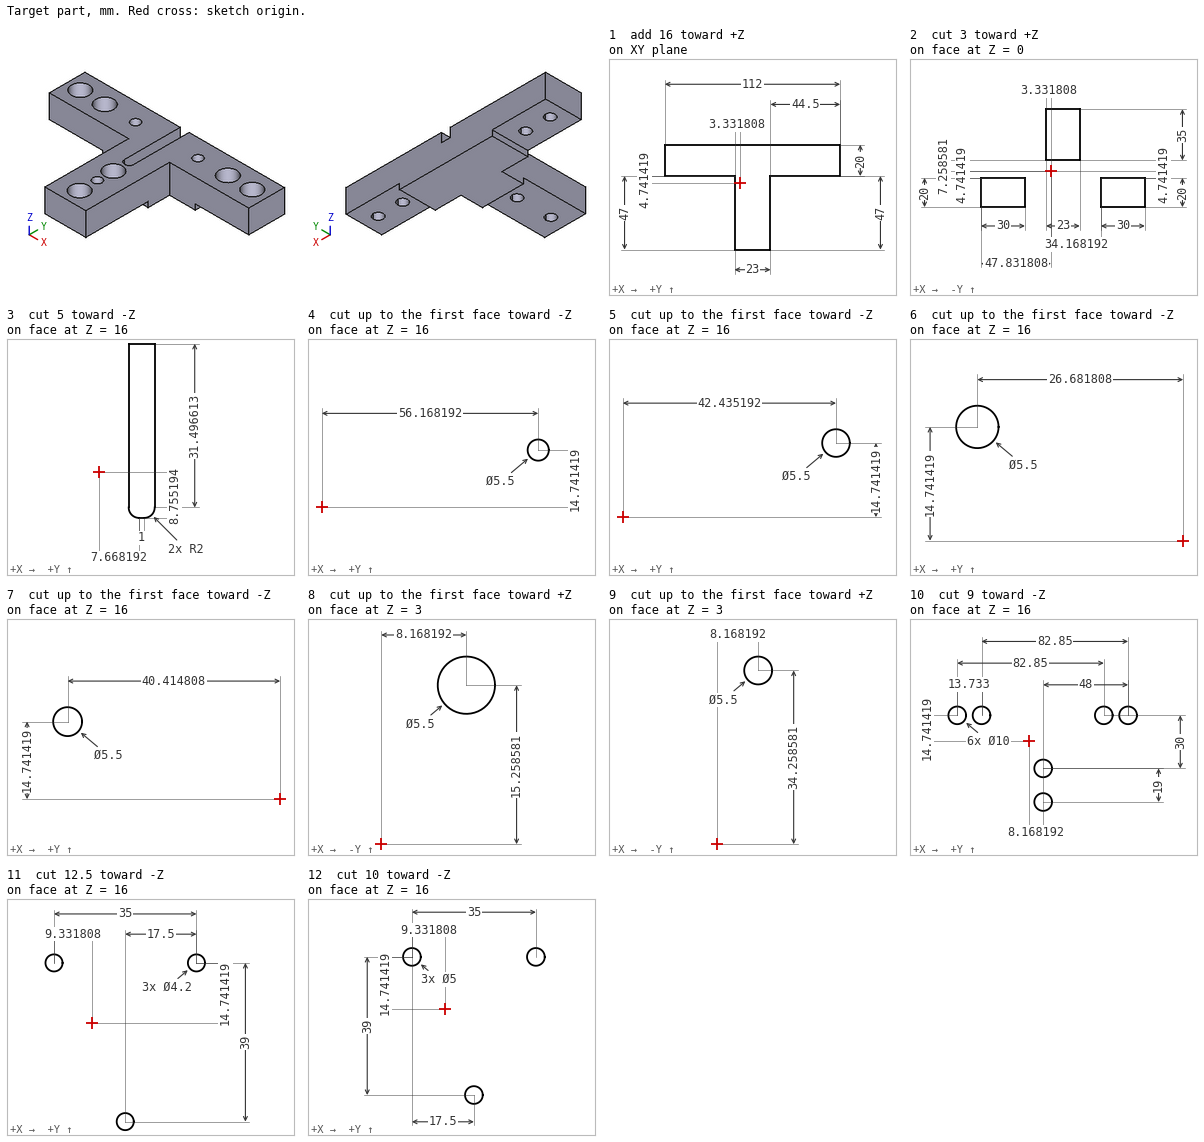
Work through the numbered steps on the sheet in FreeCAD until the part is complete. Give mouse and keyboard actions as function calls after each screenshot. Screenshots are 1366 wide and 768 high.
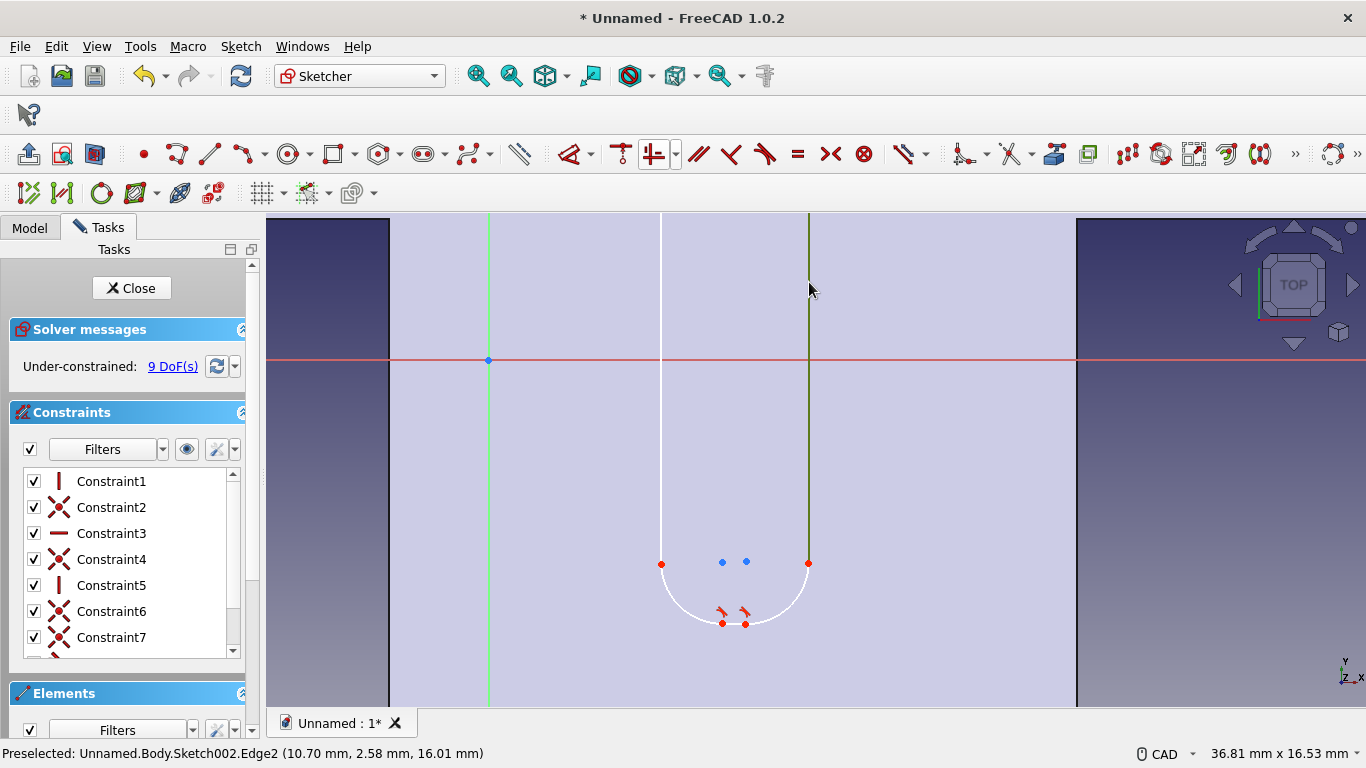
click(774, 618)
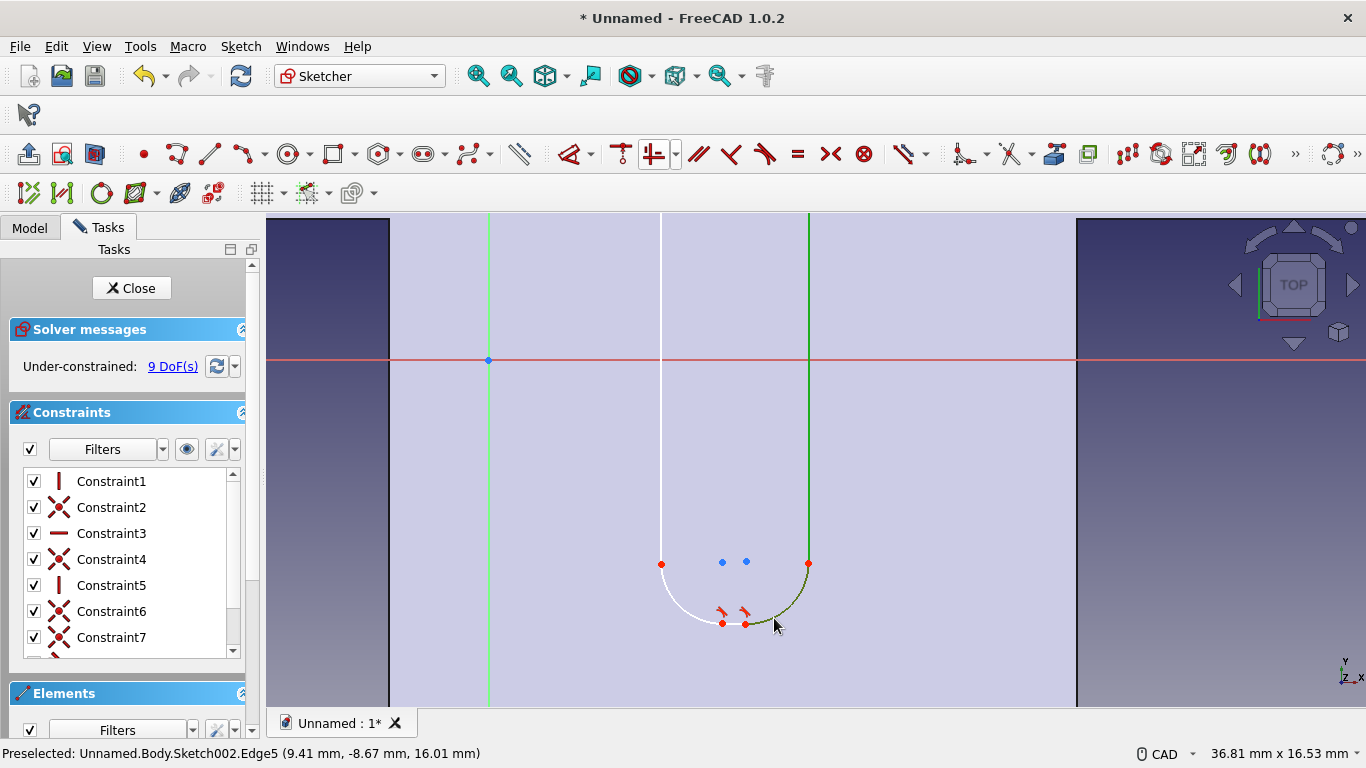
click(765, 154)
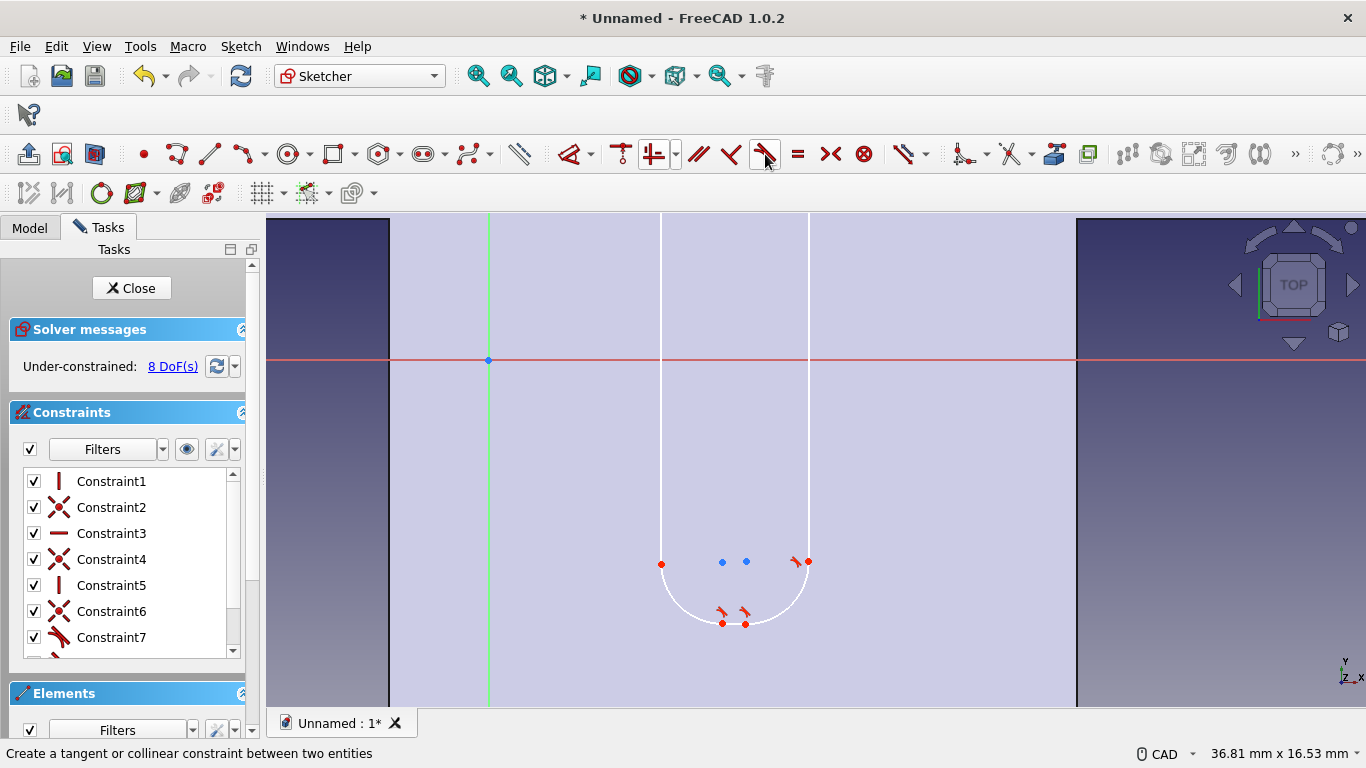
click(661, 282)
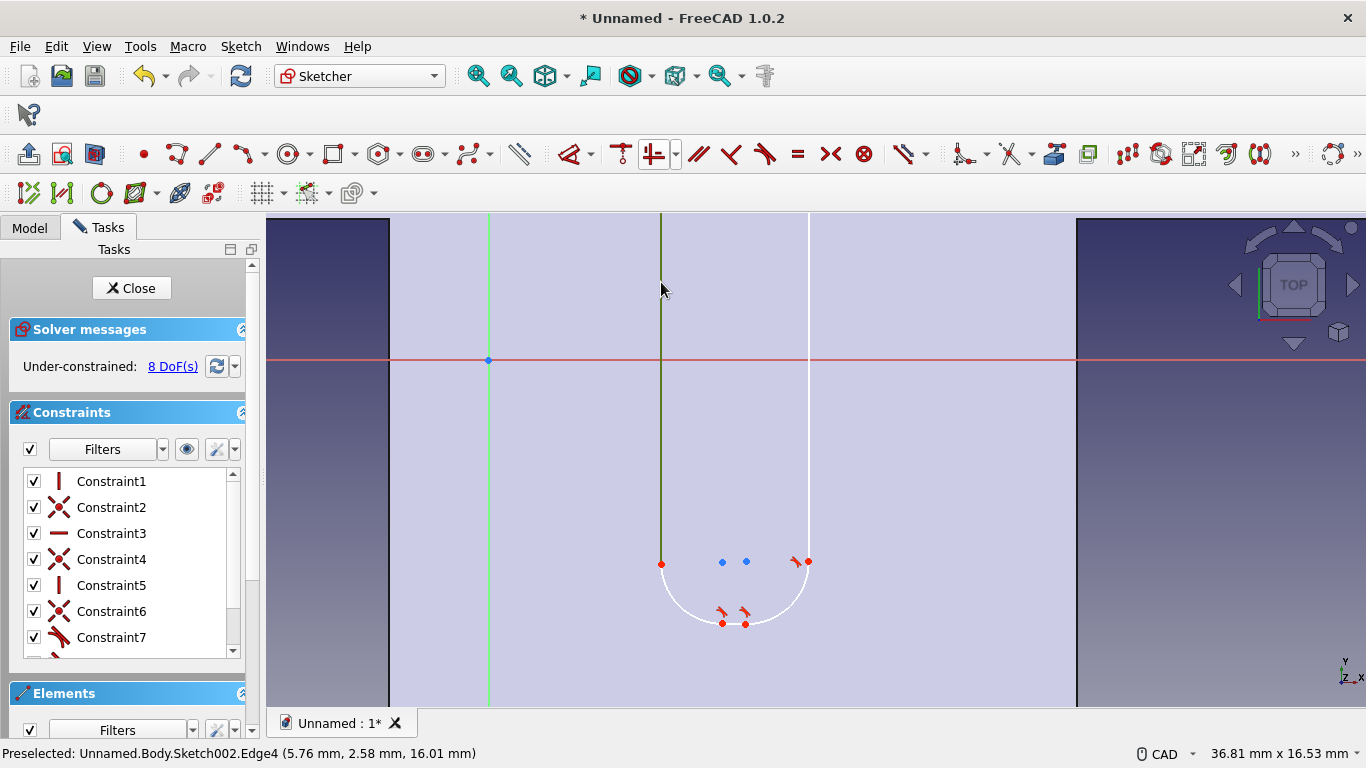
click(668, 591)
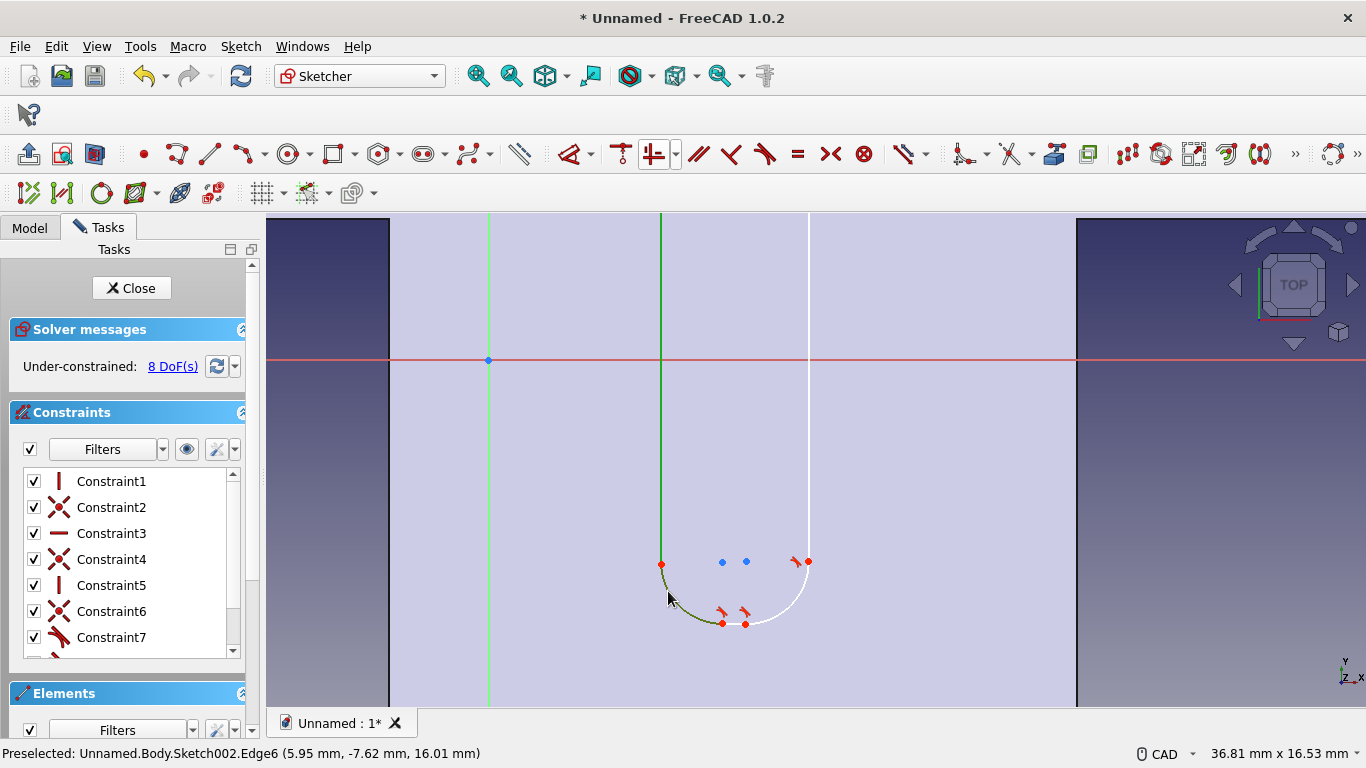
click(765, 154)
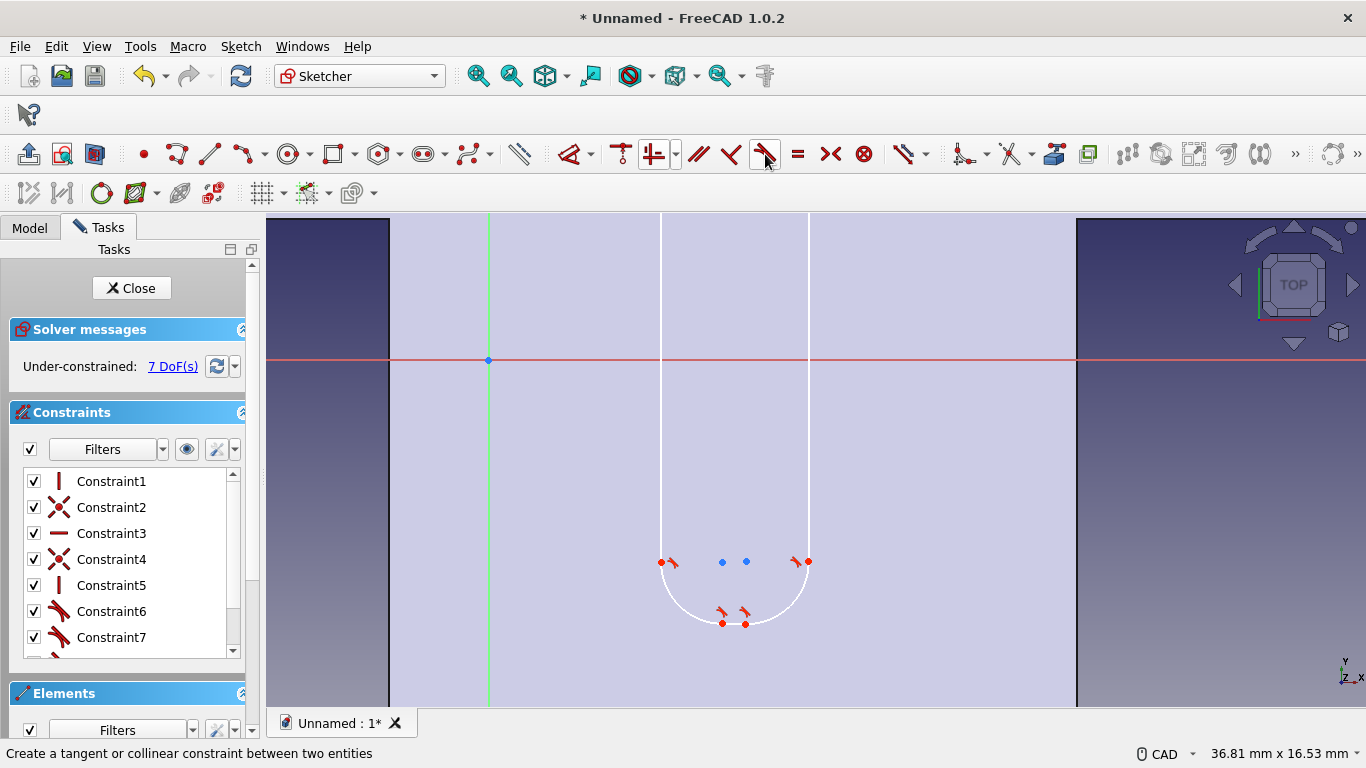
scroll(732, 624, up, 2)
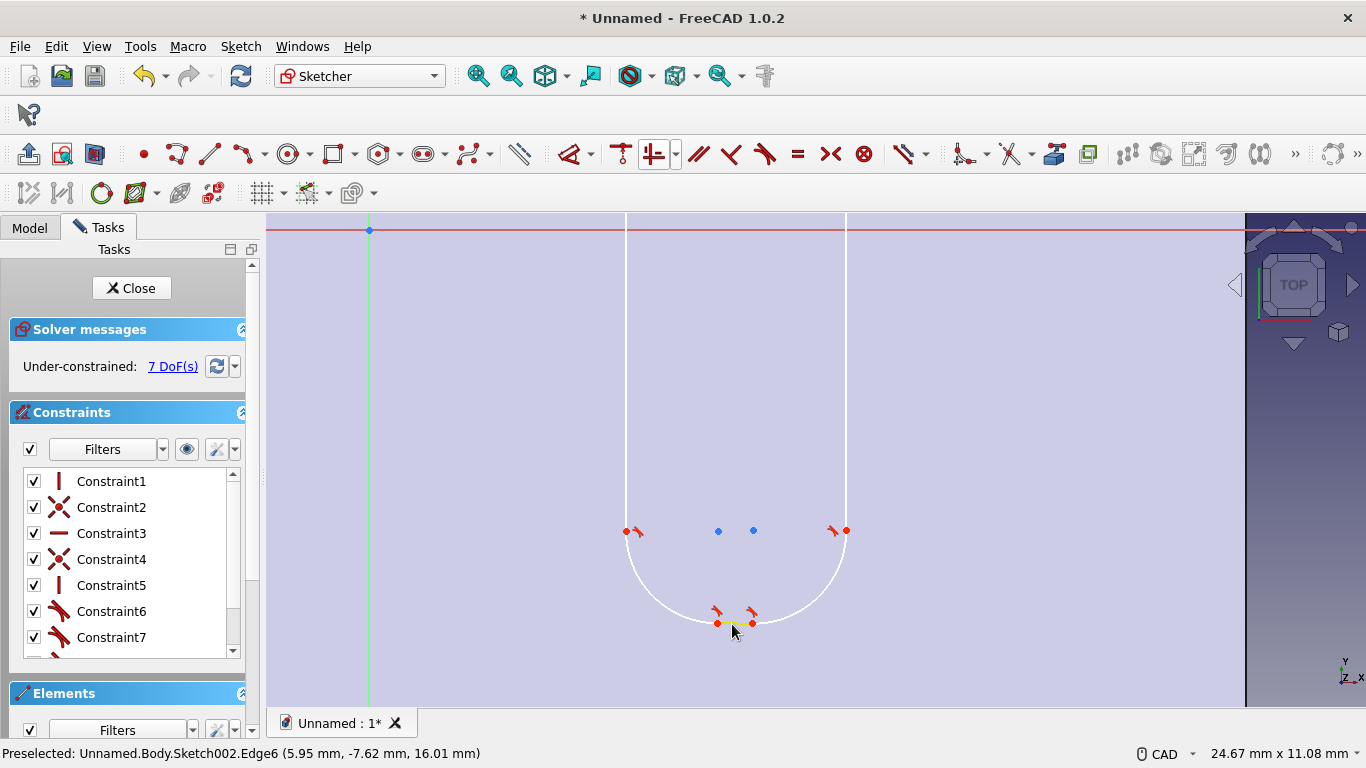
click(731, 623)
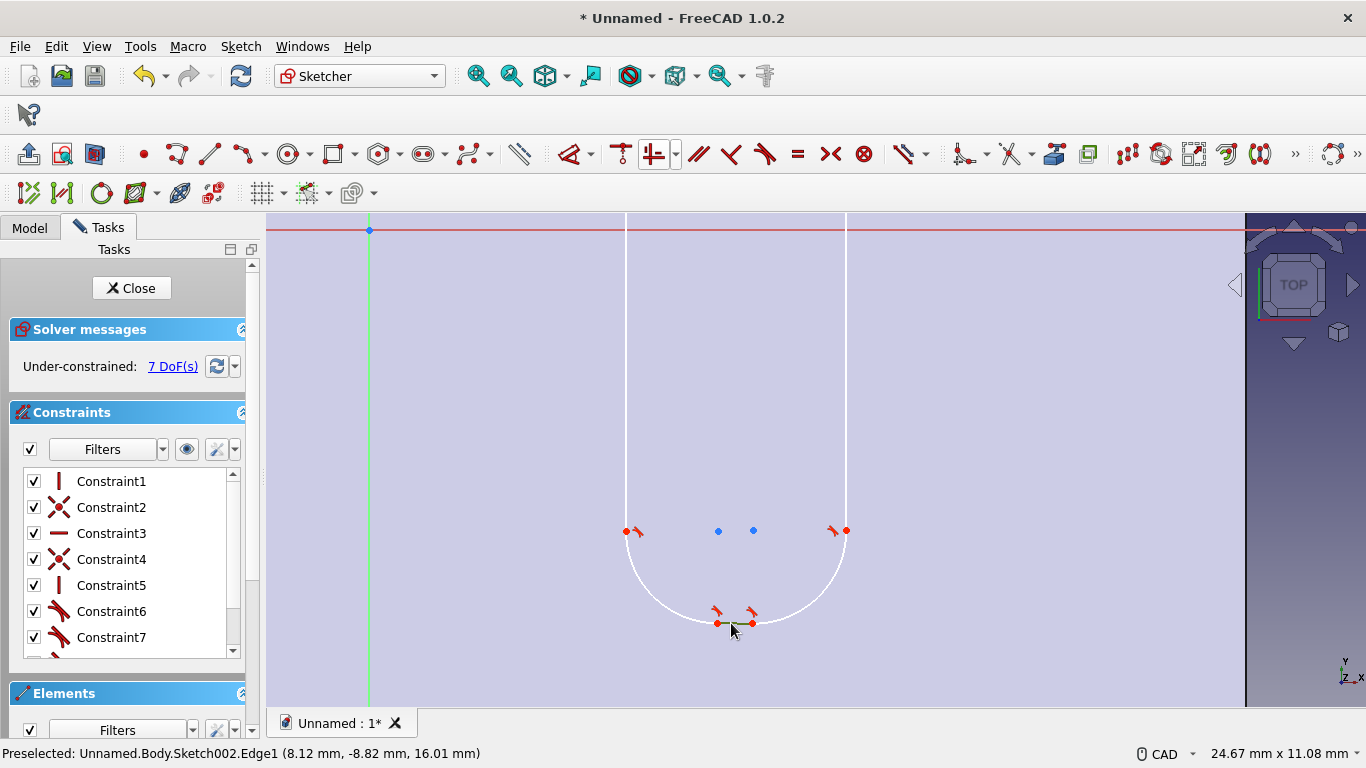
key(h)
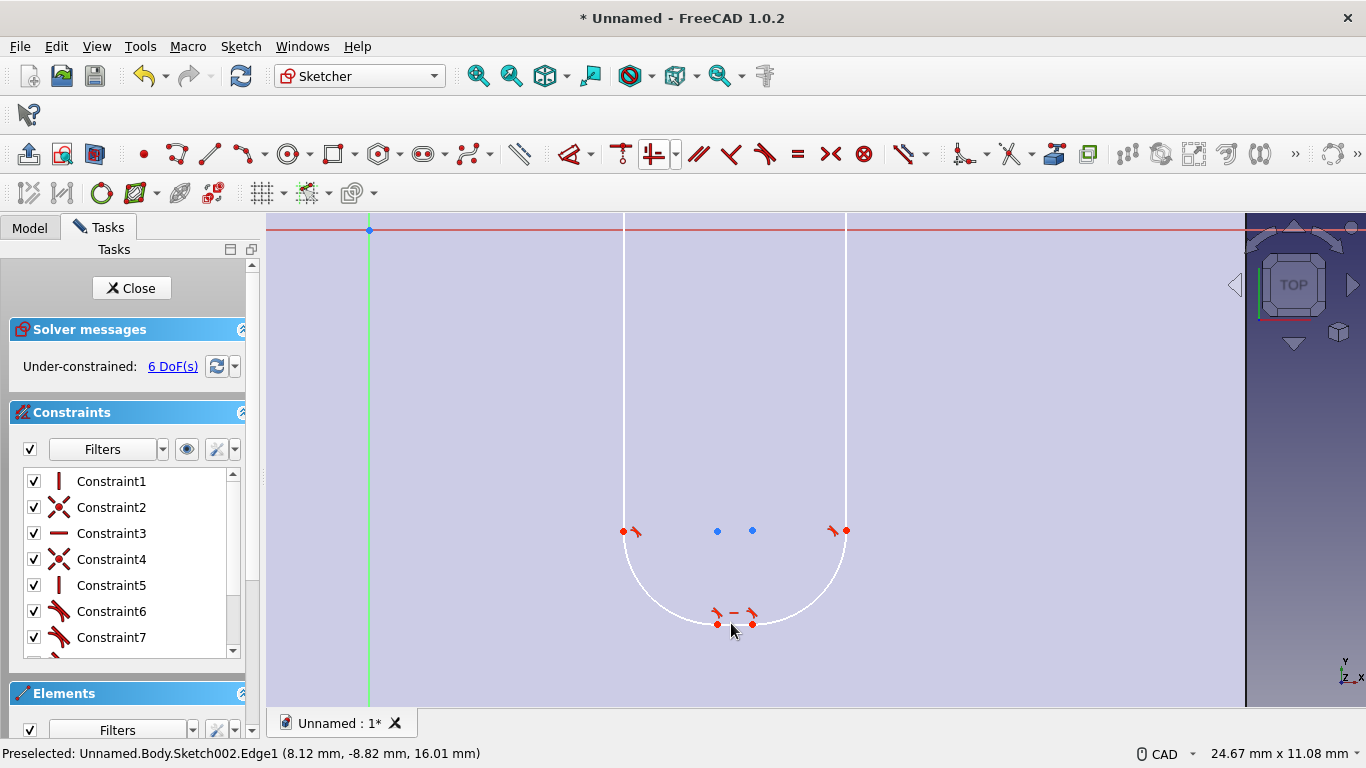
scroll(783, 608, down, 8)